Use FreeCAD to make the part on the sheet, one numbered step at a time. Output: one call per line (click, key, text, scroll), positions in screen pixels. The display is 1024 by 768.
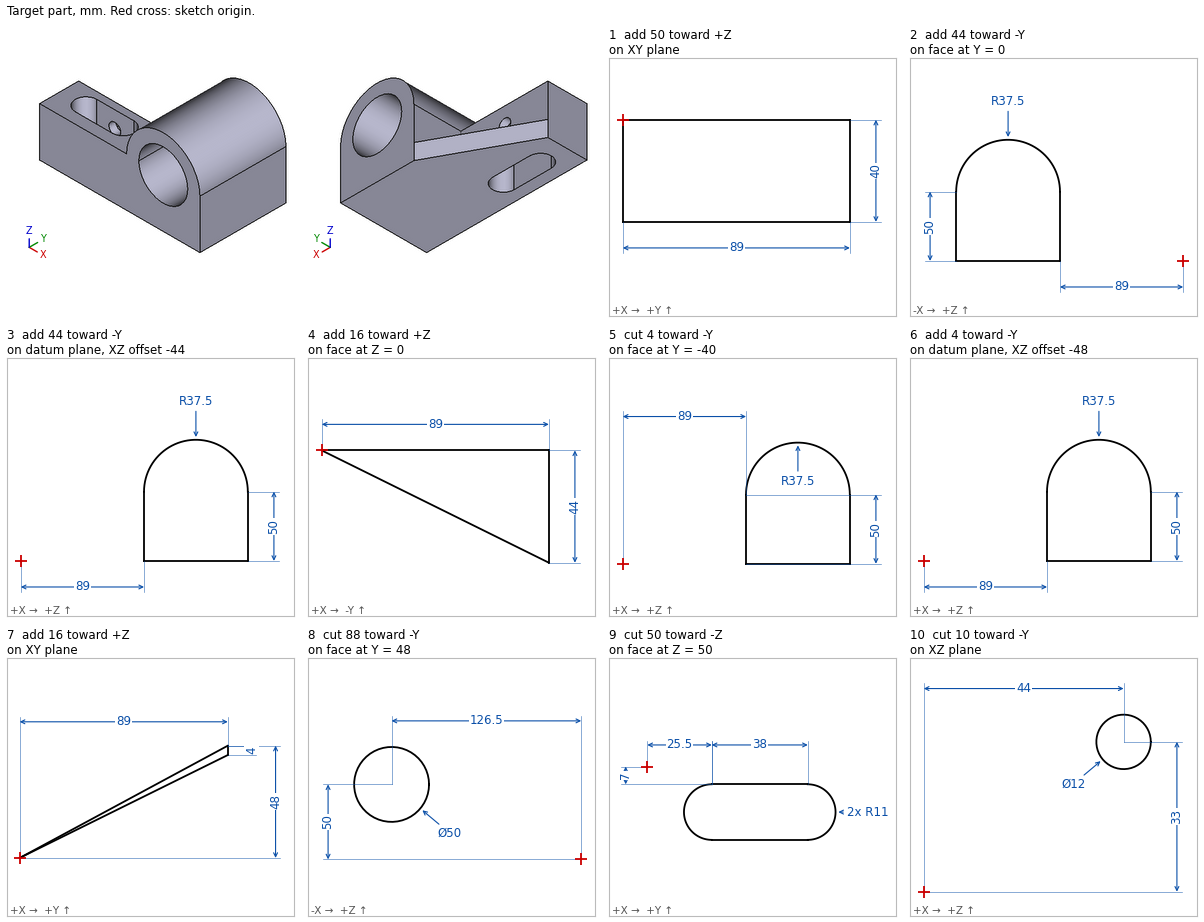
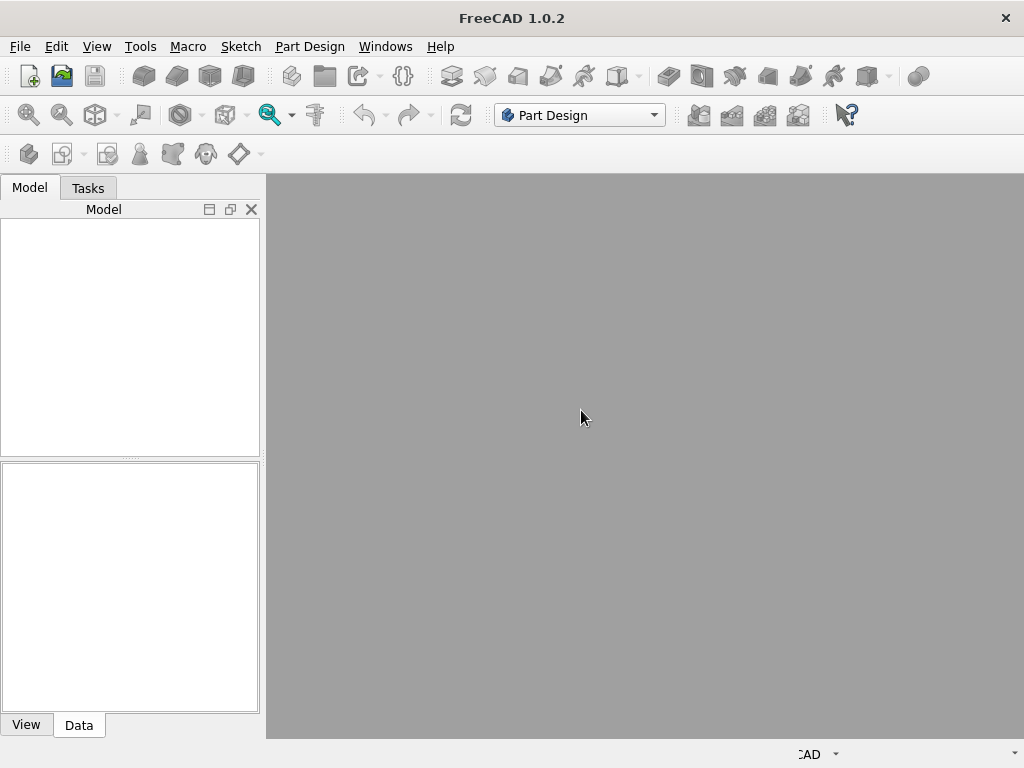
key(ctrl+n)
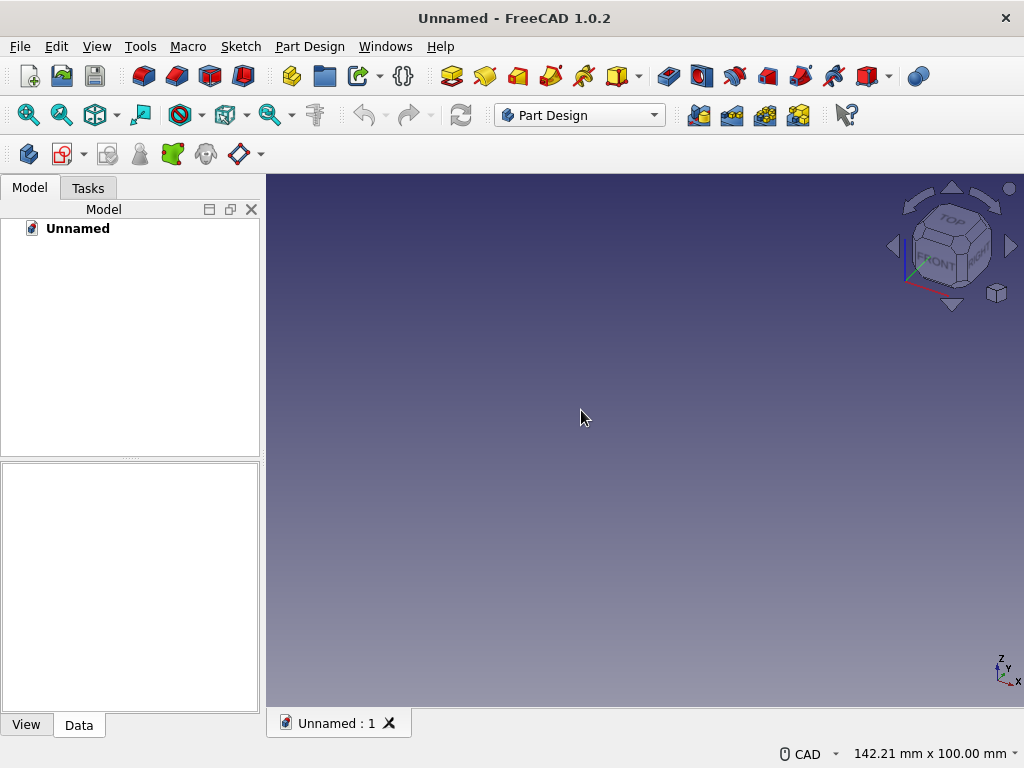
click(62, 154)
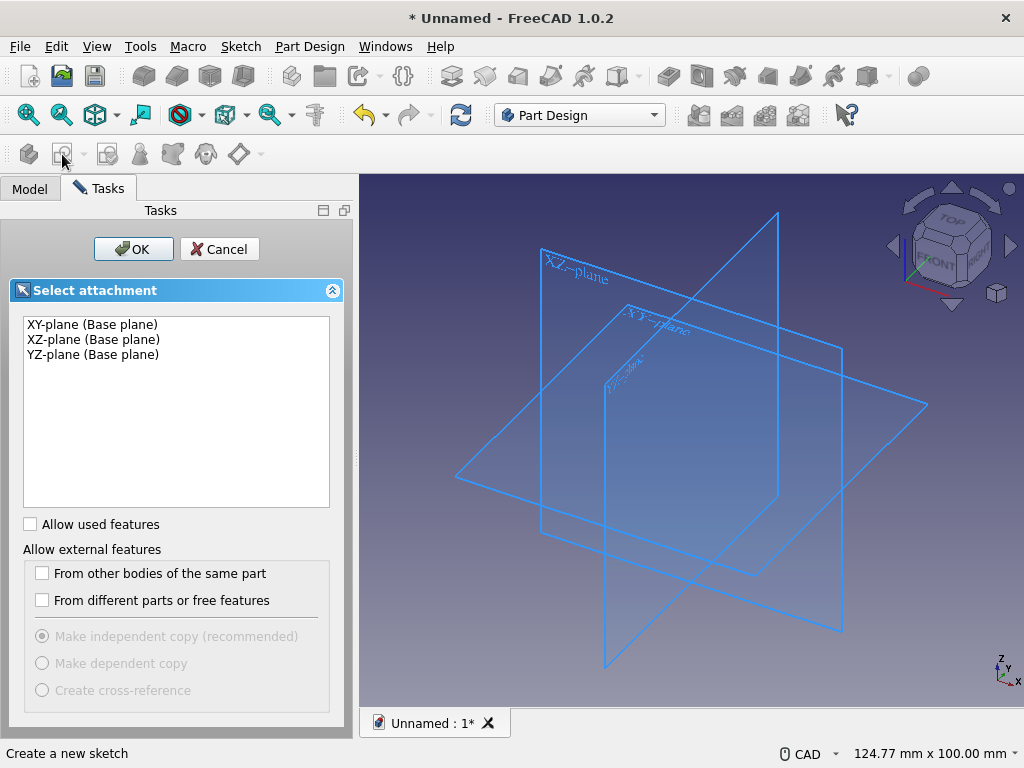
click(84, 324)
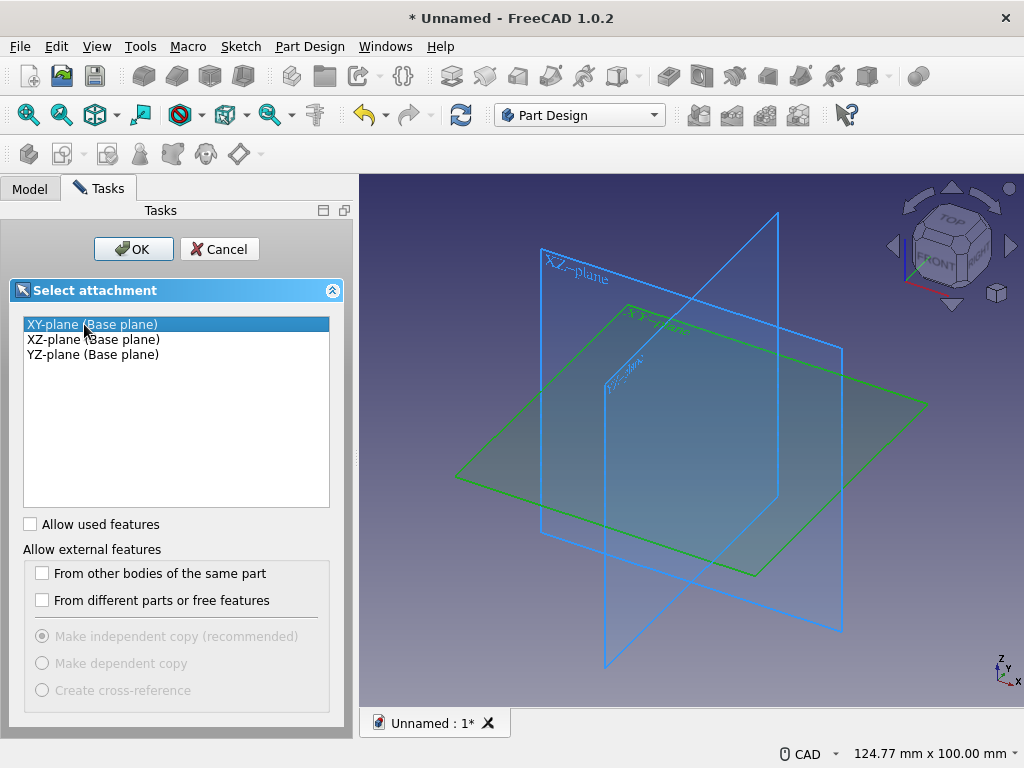
click(134, 249)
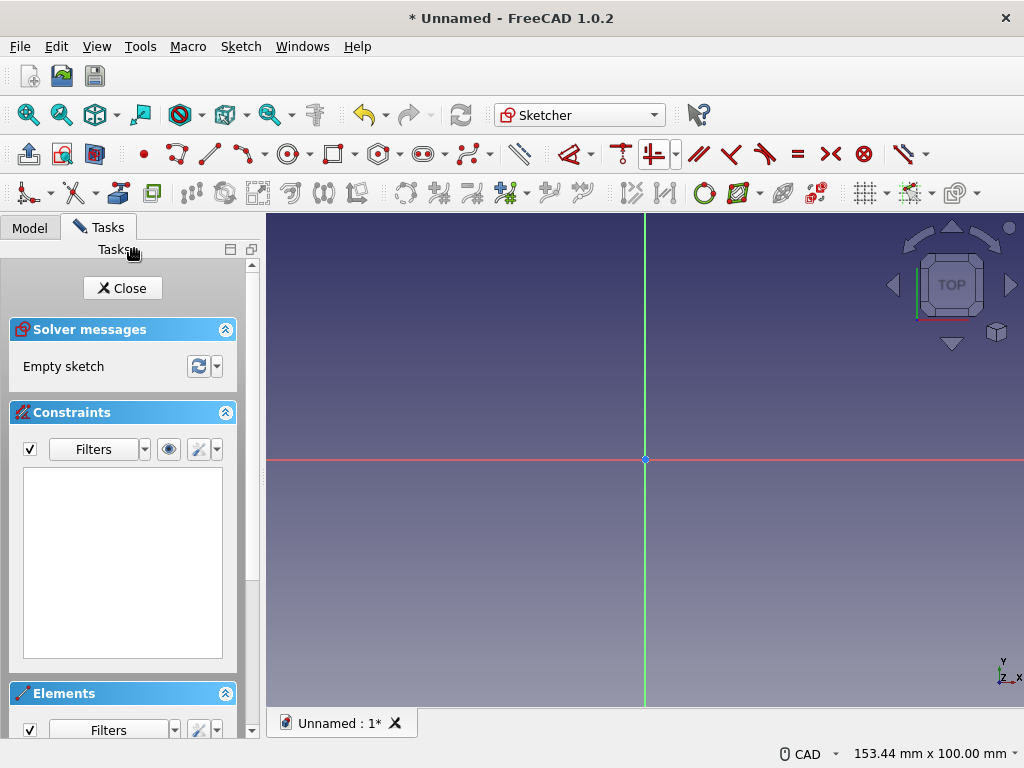
scroll(294, 259, down, 2)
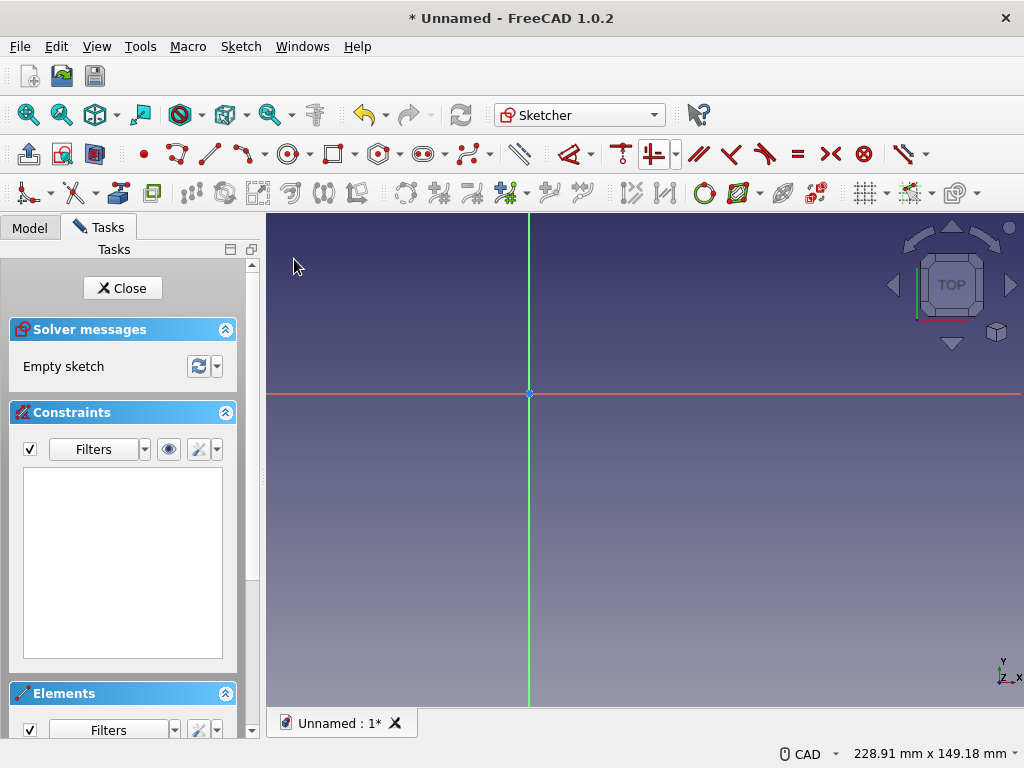
scroll(859, 460, up, 2)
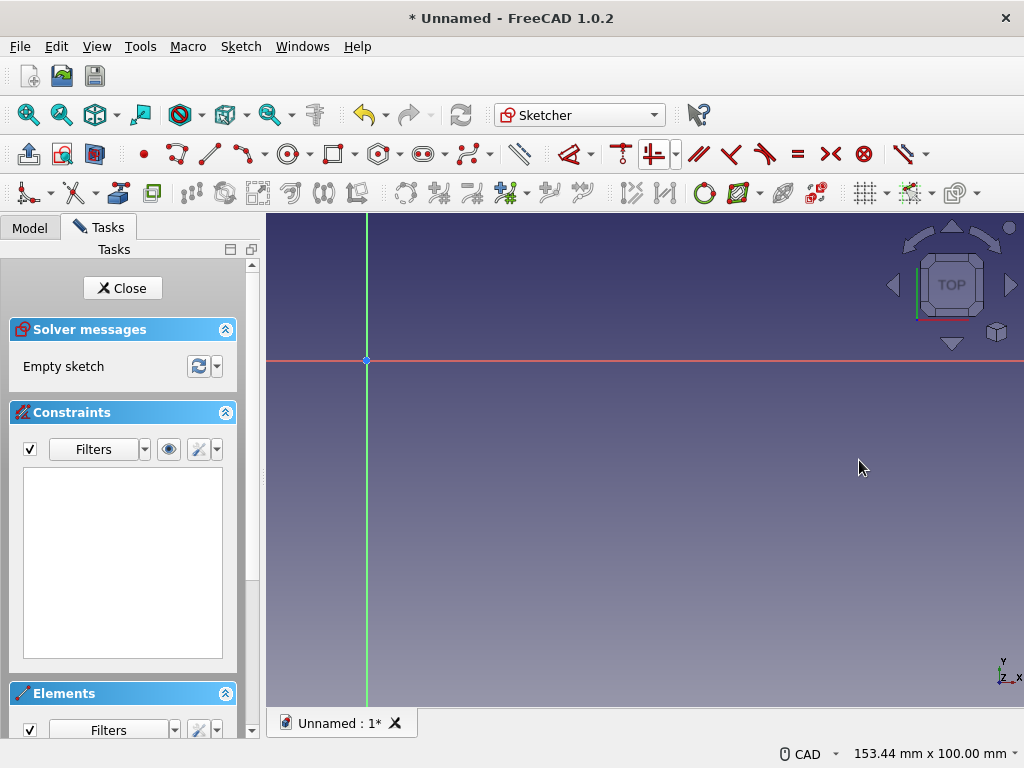
click(332, 154)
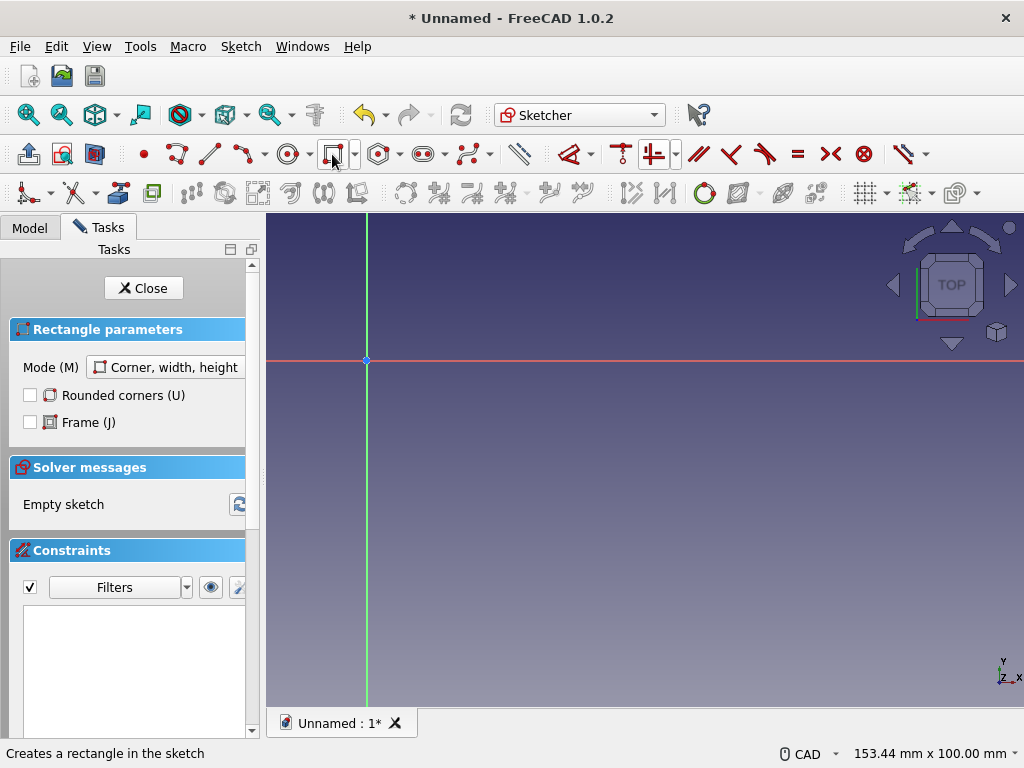
click(367, 361)
move(806, 559)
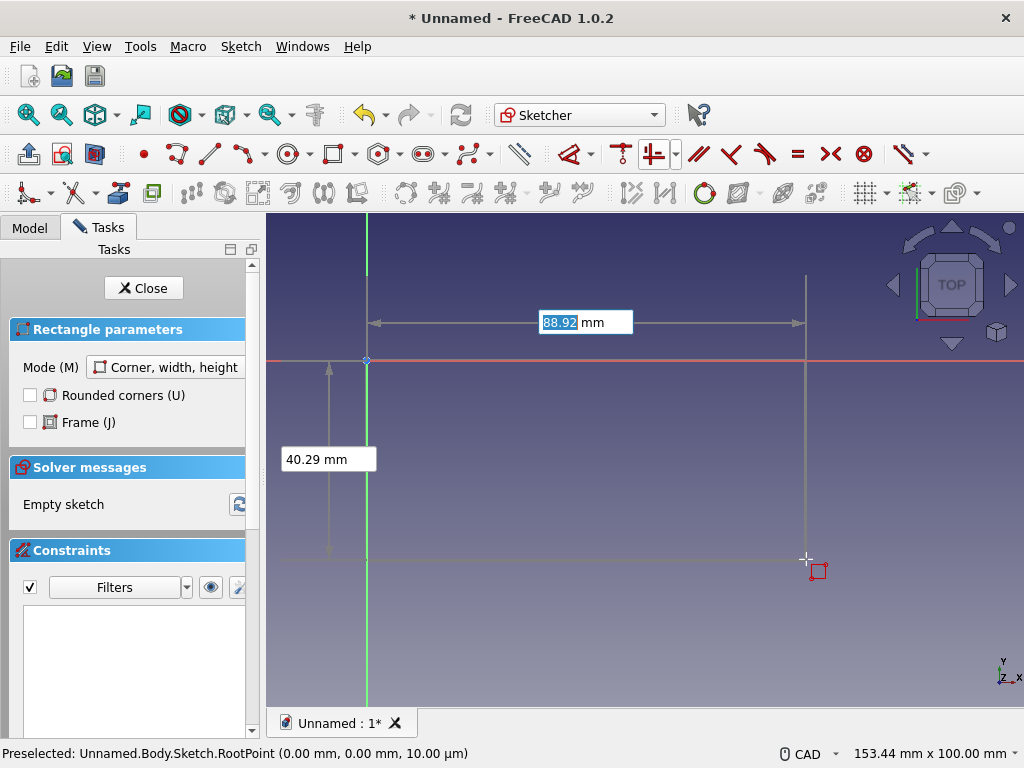
text(89)
key(Tab)
text(40)
key(Return)
key(Escape)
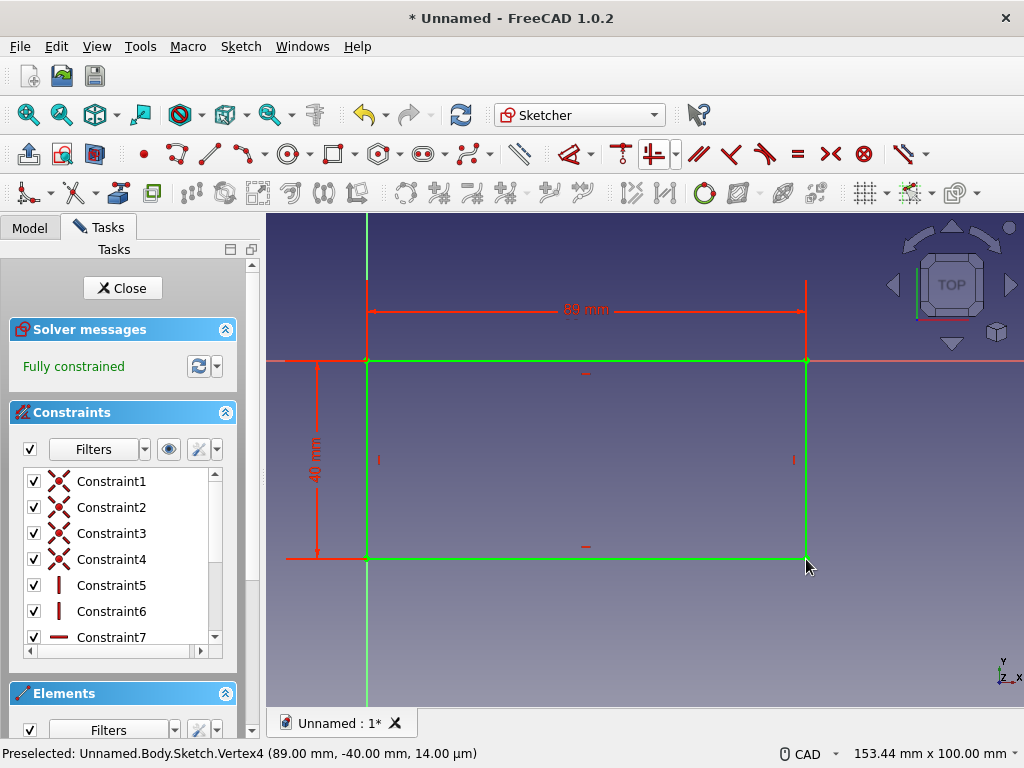
click(123, 288)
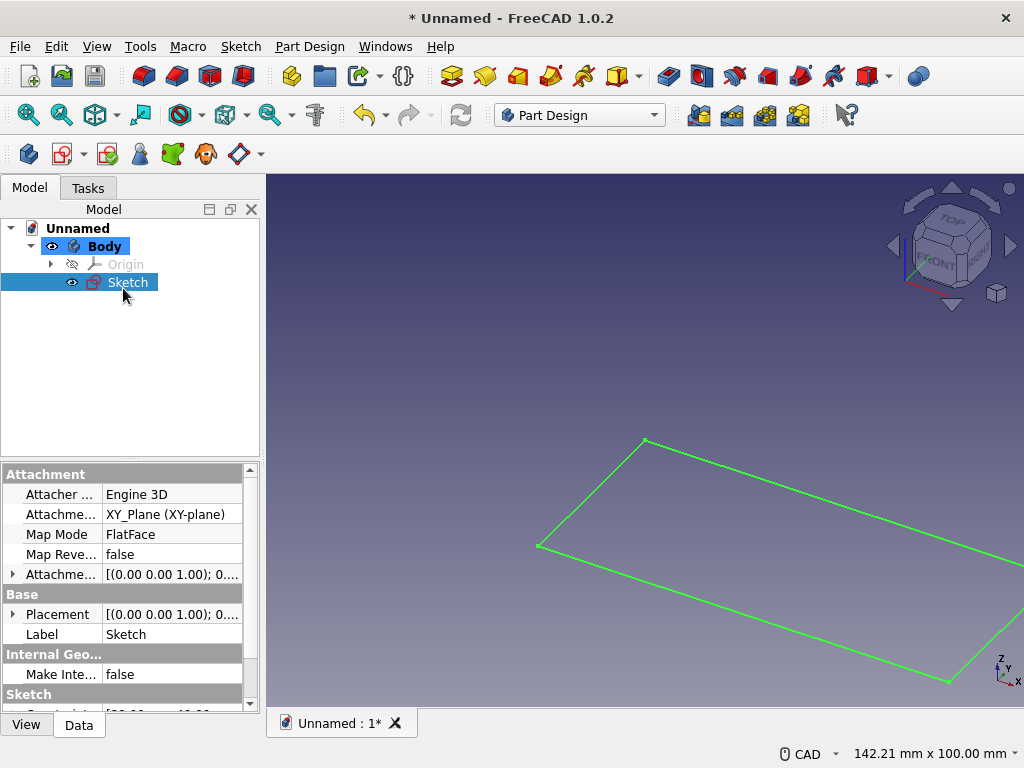
click(452, 76)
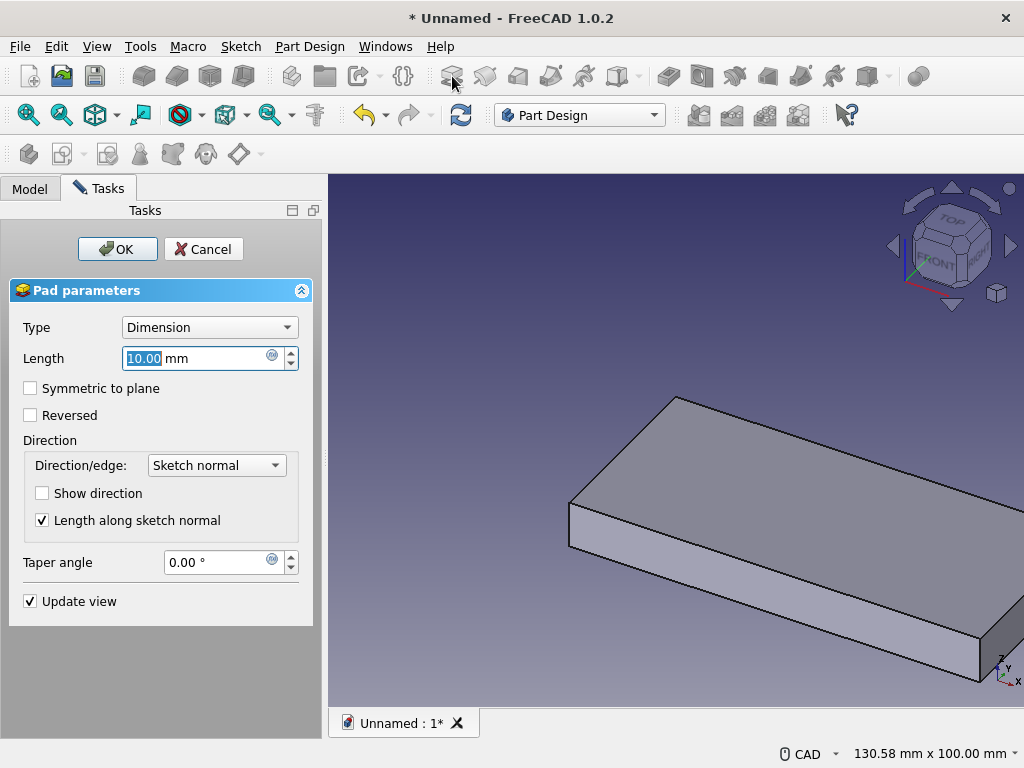
text(50)
key(Tab)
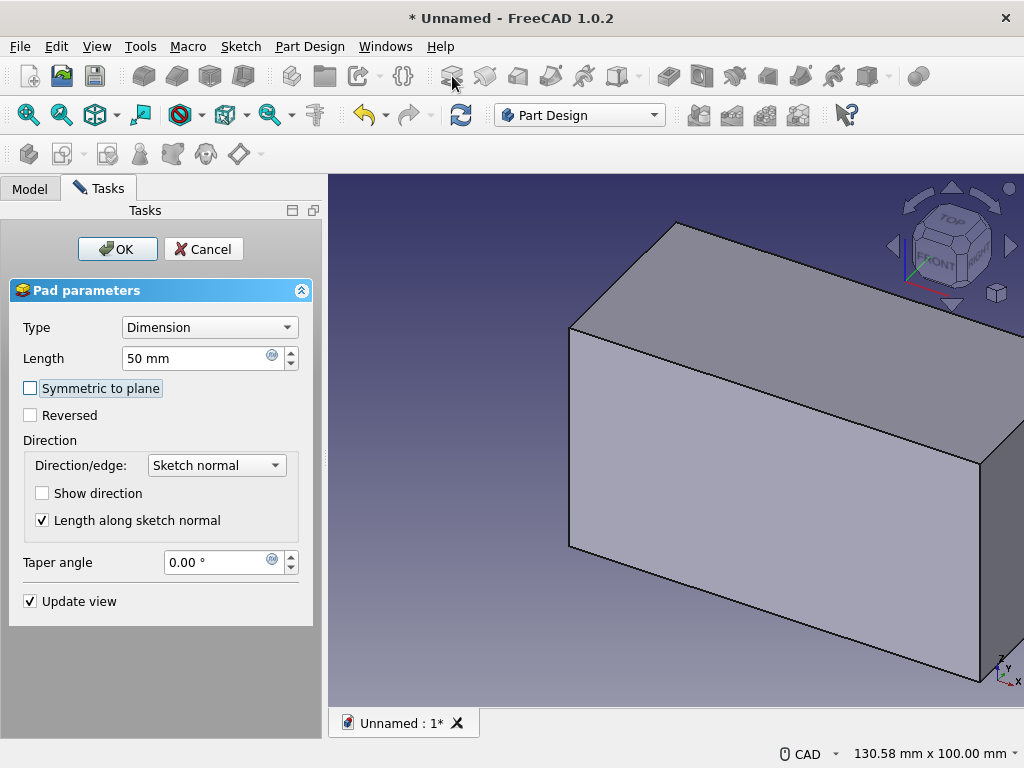
click(118, 249)